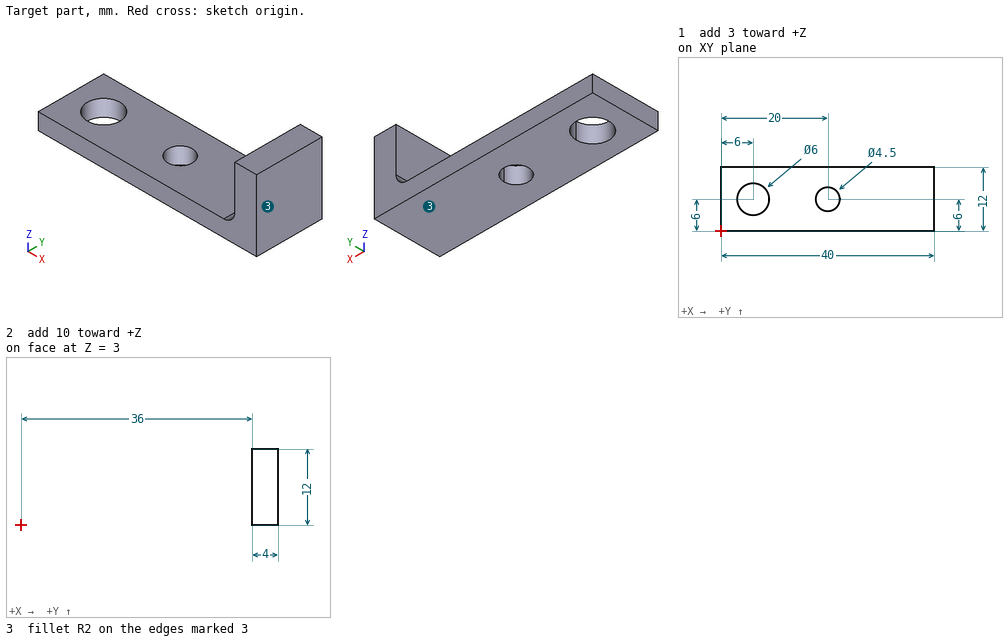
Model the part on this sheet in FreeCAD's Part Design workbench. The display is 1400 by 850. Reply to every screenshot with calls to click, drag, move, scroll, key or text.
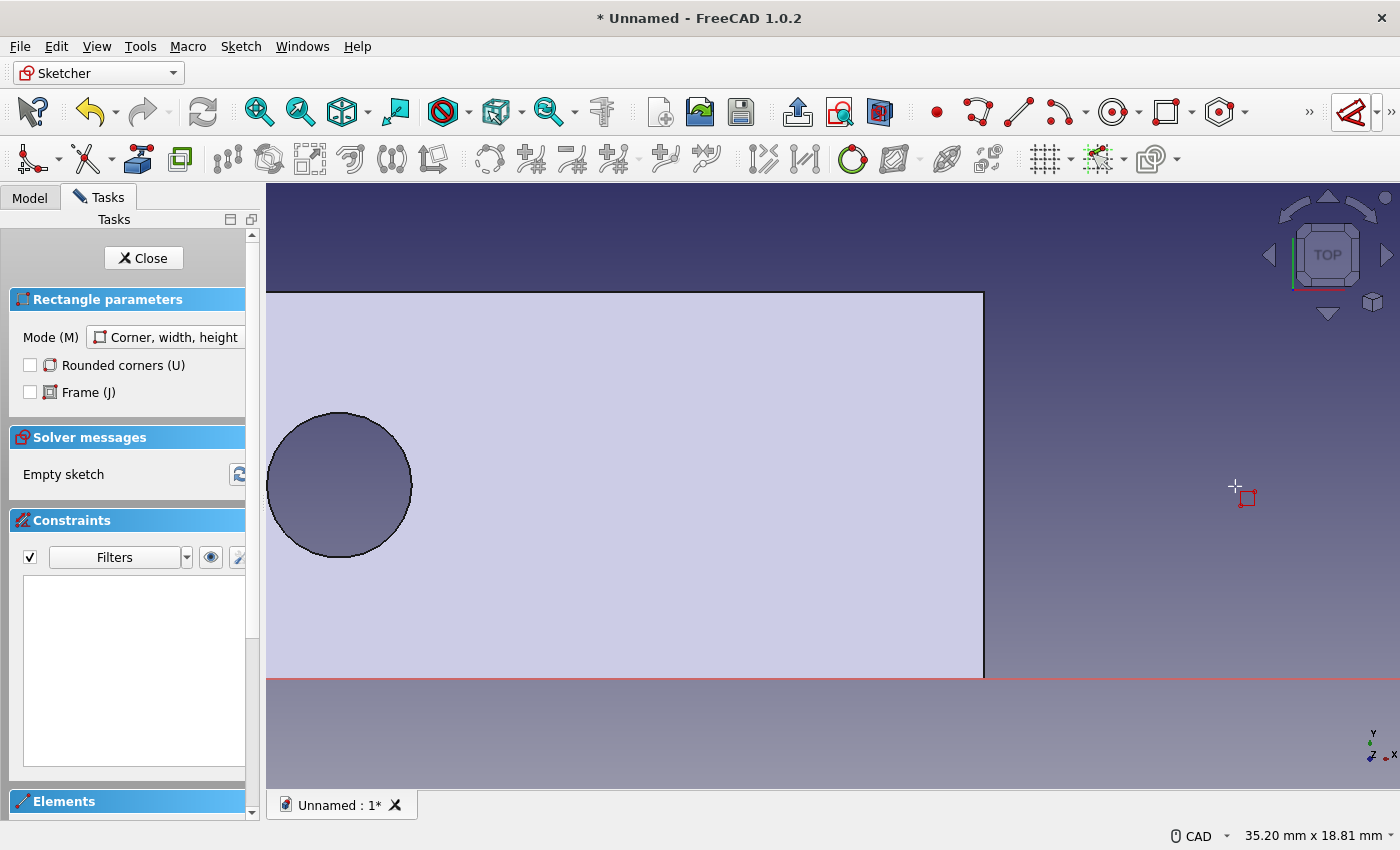
click(855, 292)
click(984, 679)
key(Escape)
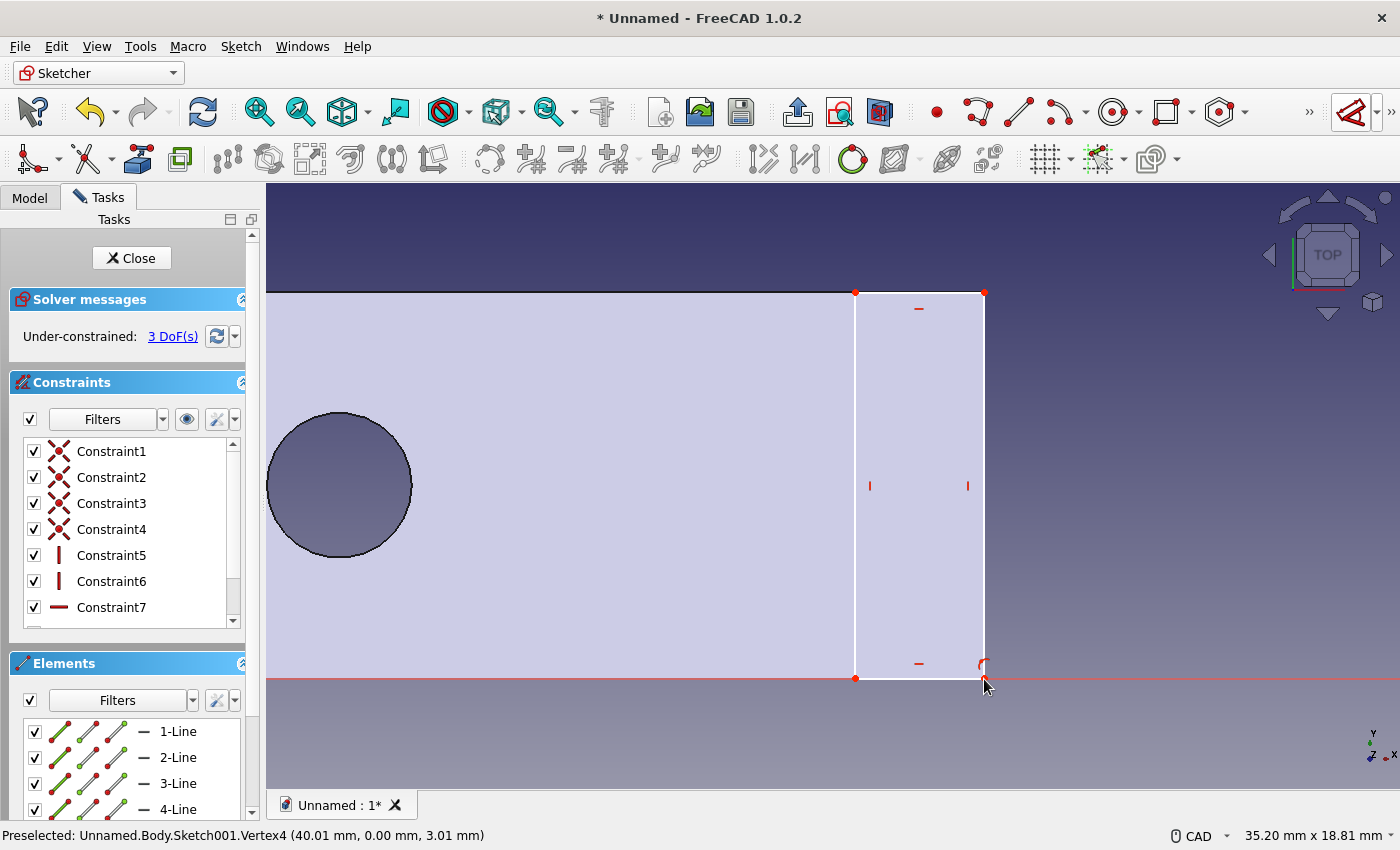
click(894, 679)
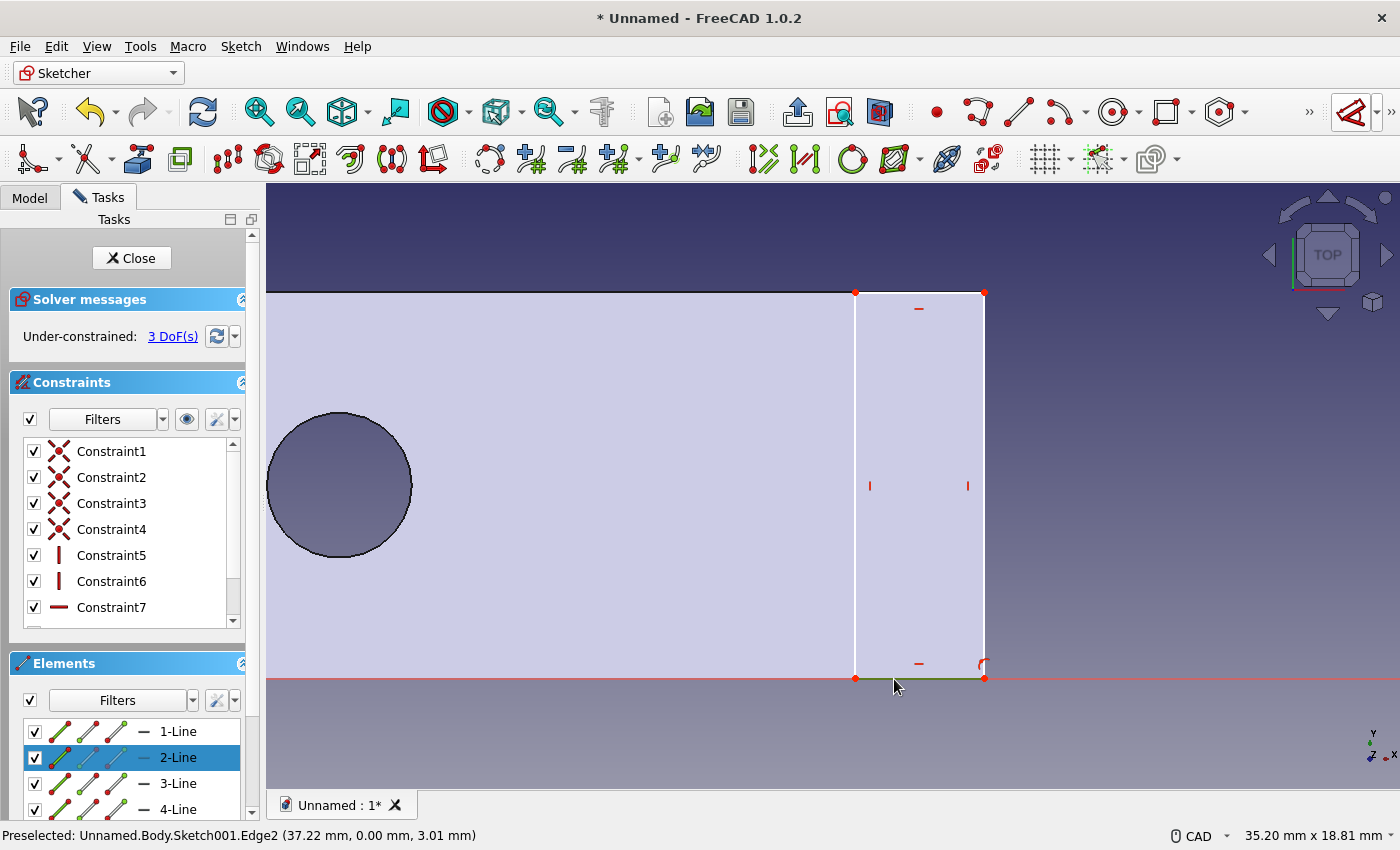
key(l)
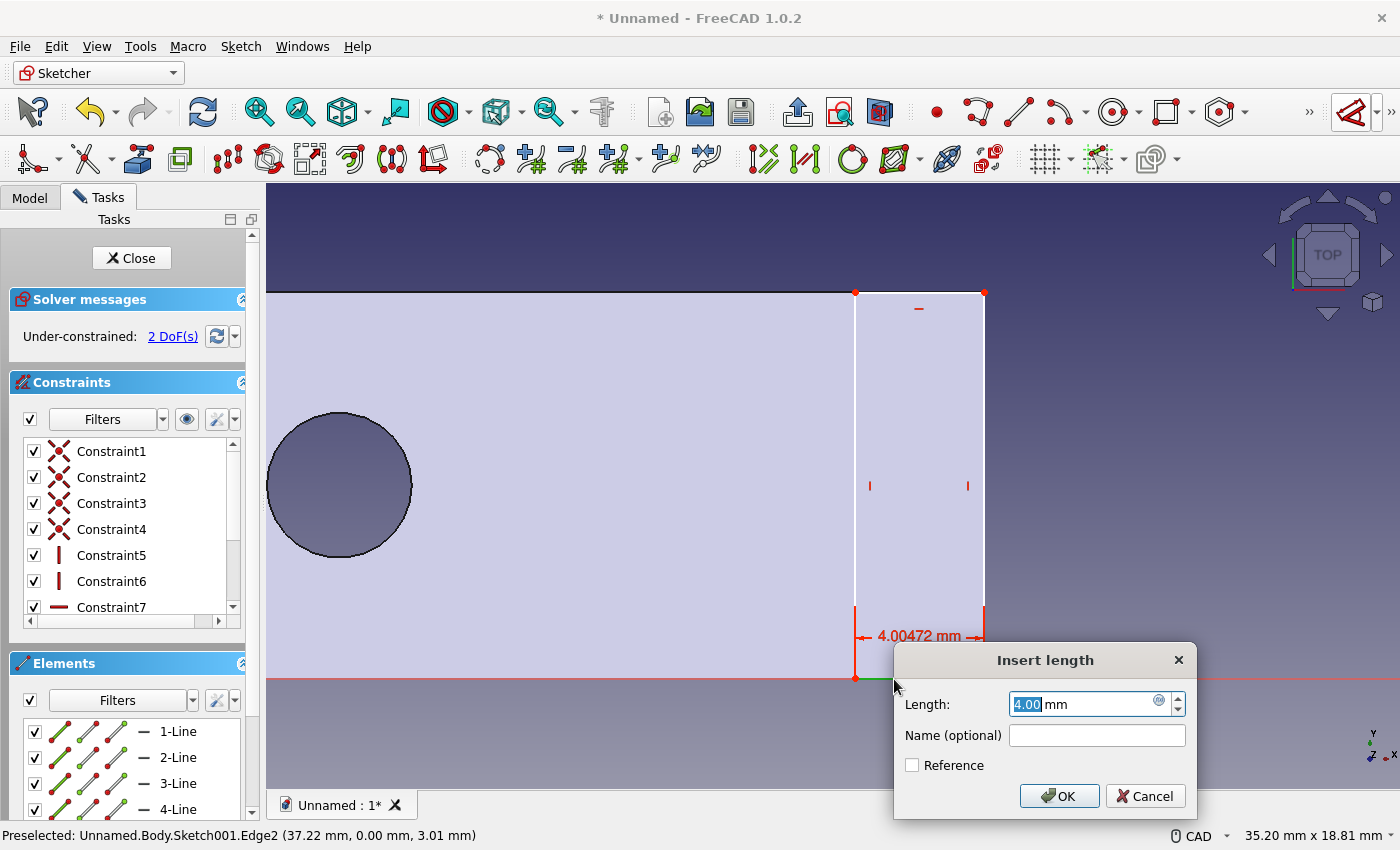
text(4)
key(Return)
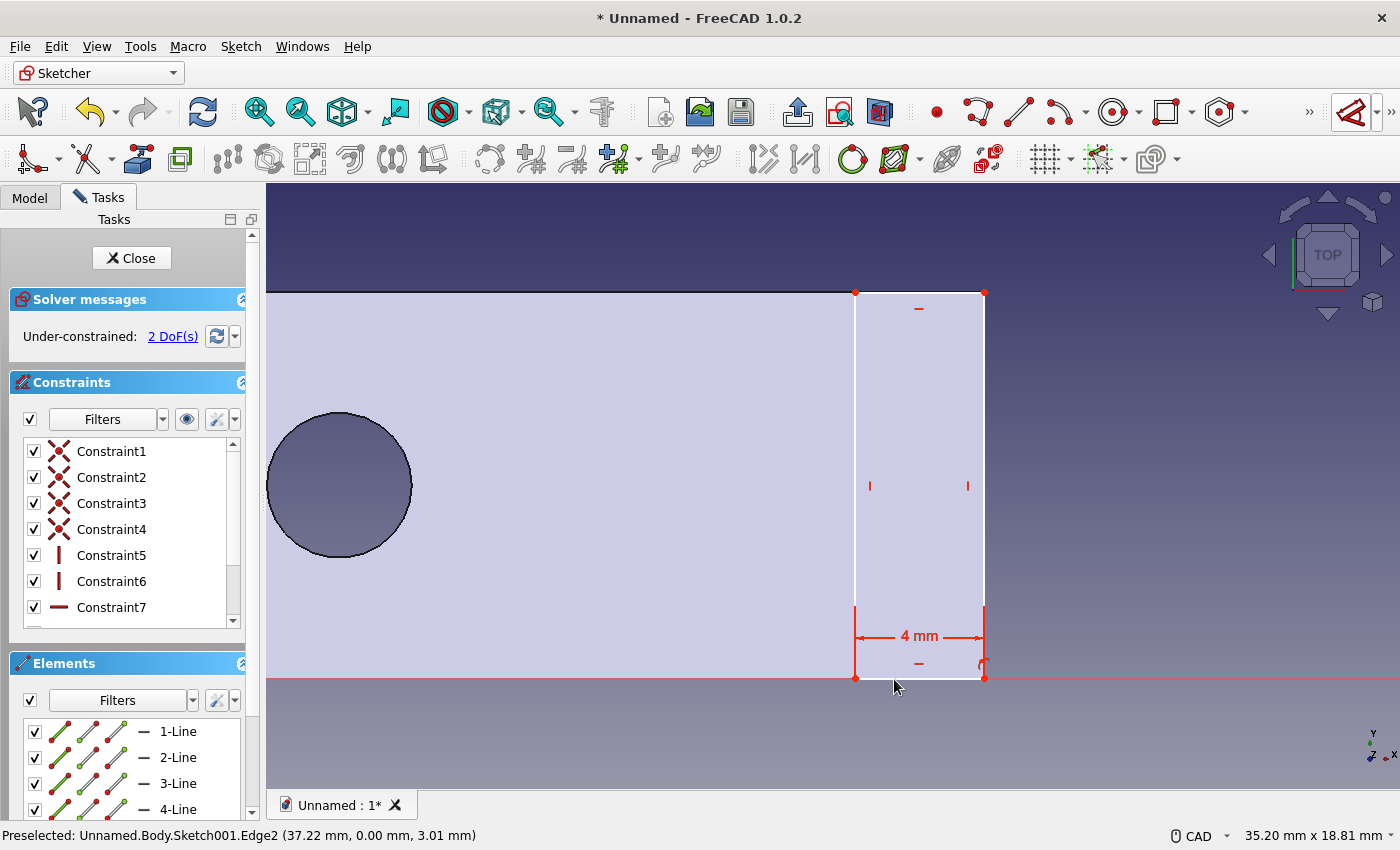
click(855, 409)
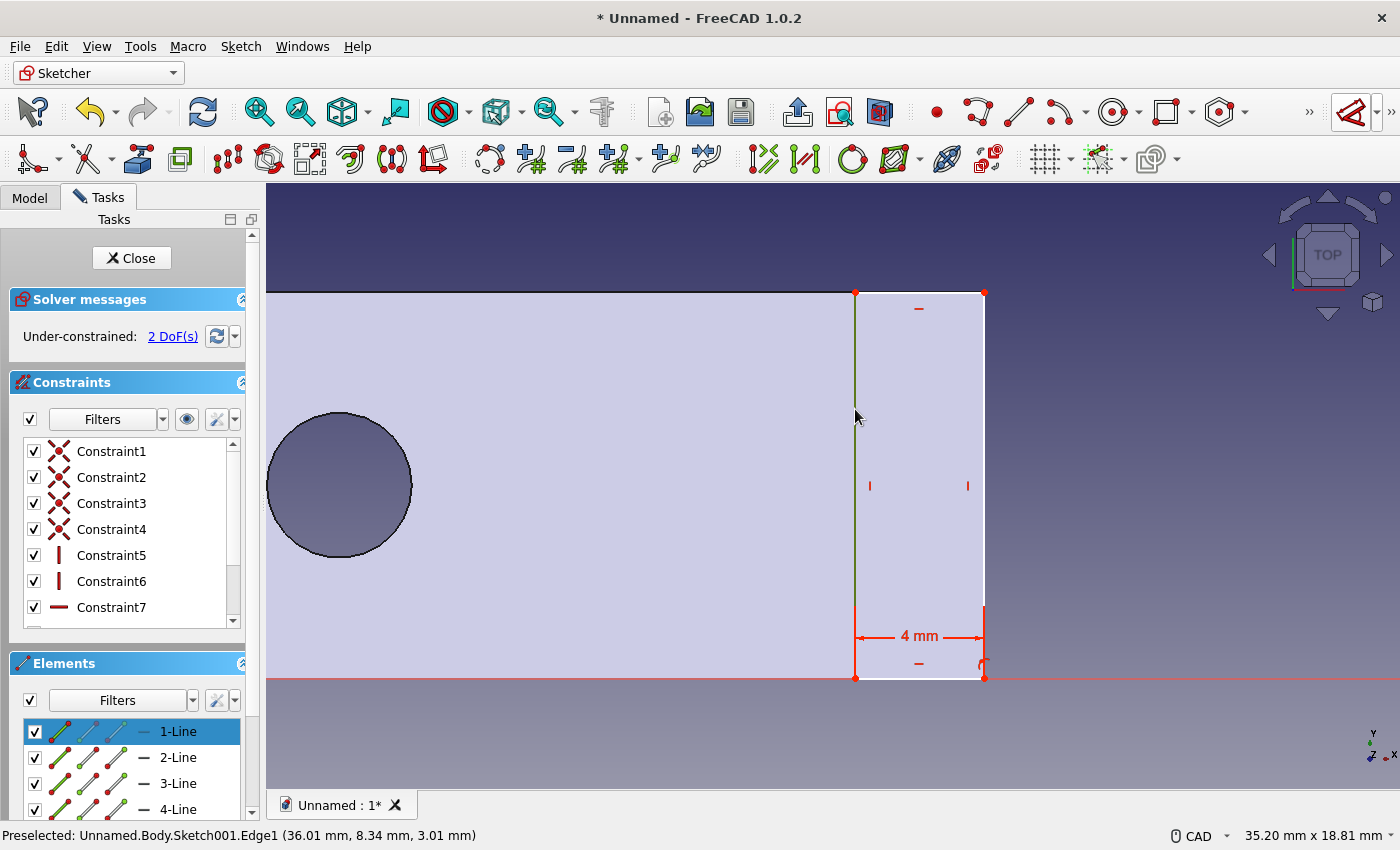
key(i)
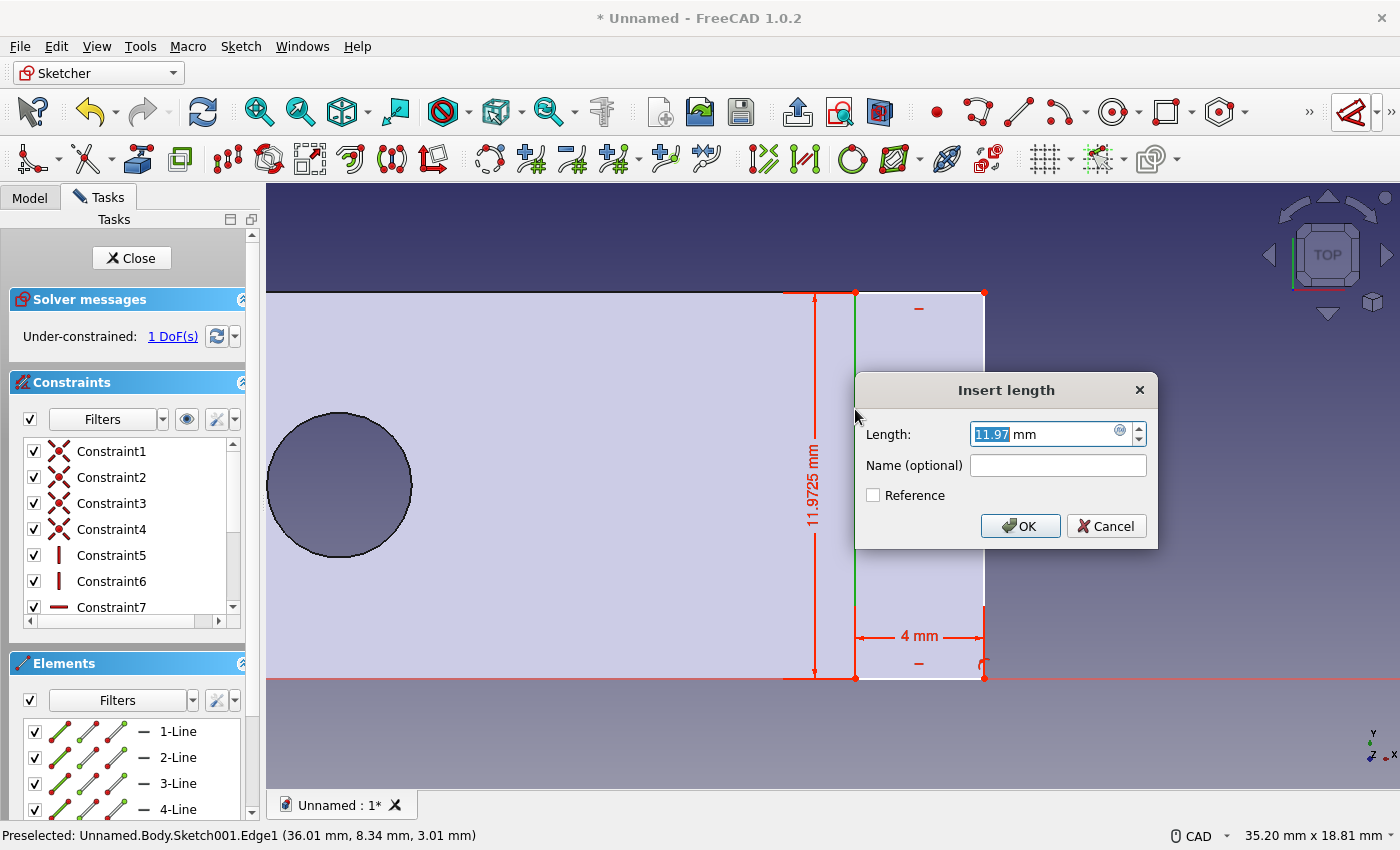
text(12)
key(Return)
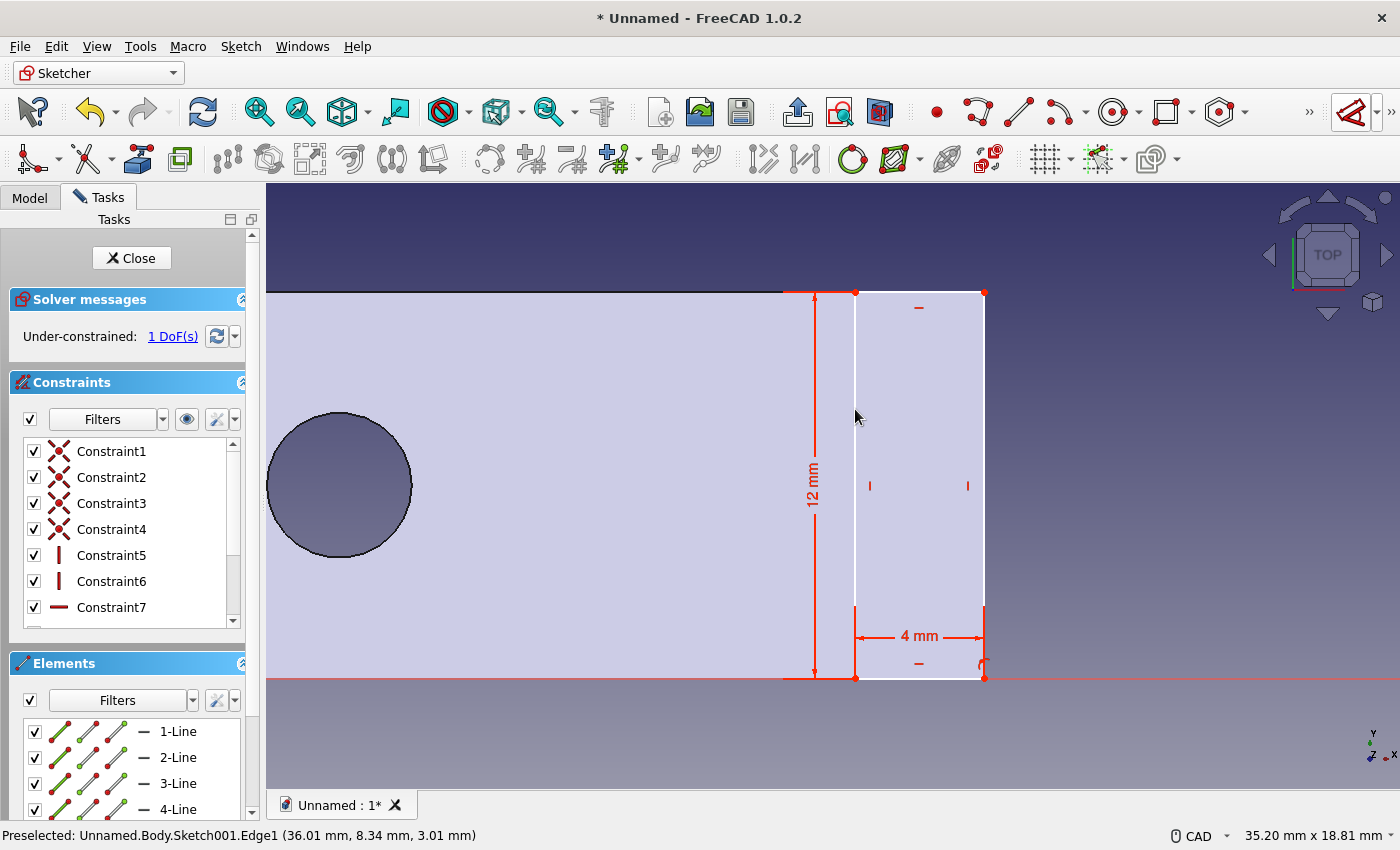
click(855, 292)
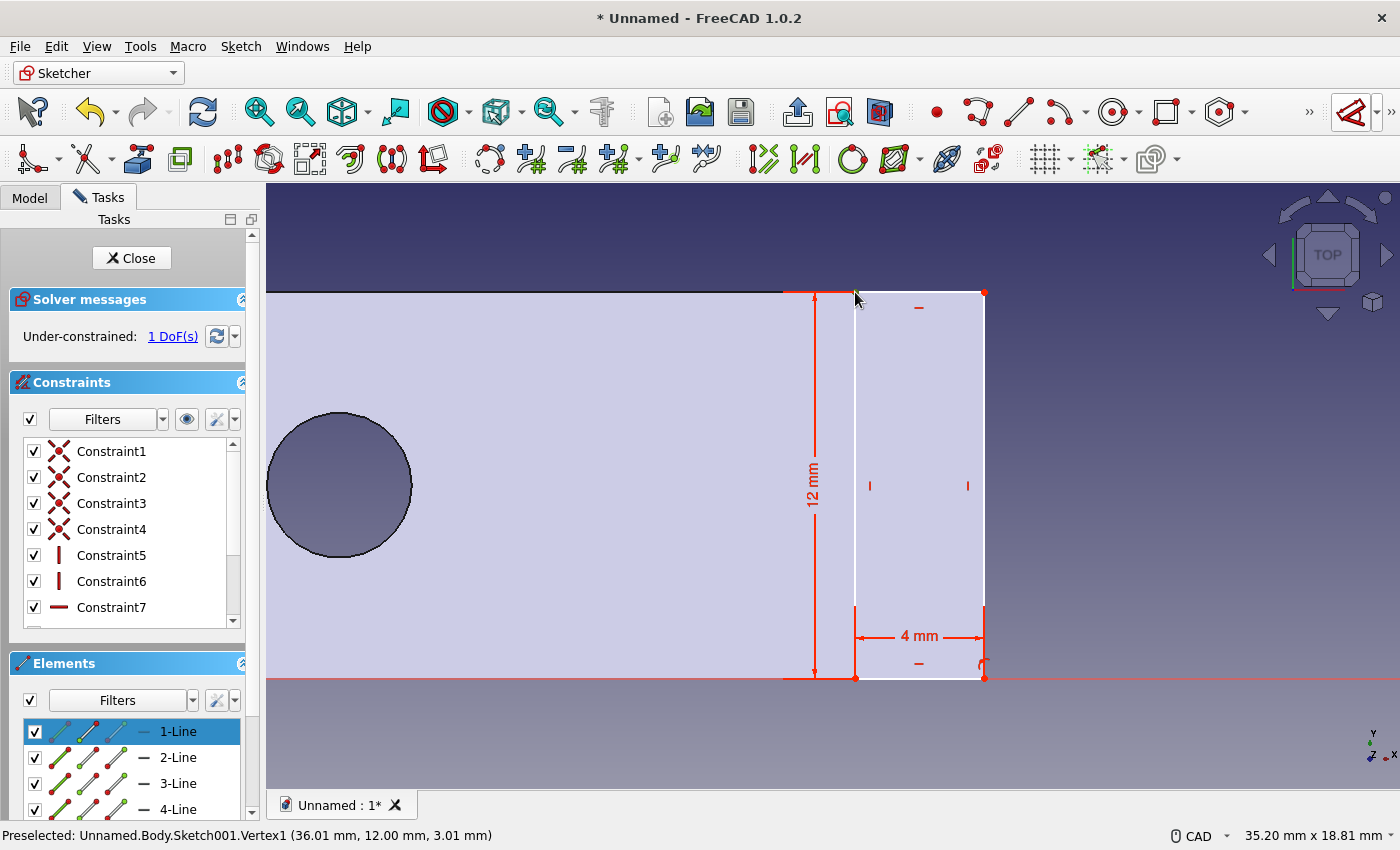
key(l)